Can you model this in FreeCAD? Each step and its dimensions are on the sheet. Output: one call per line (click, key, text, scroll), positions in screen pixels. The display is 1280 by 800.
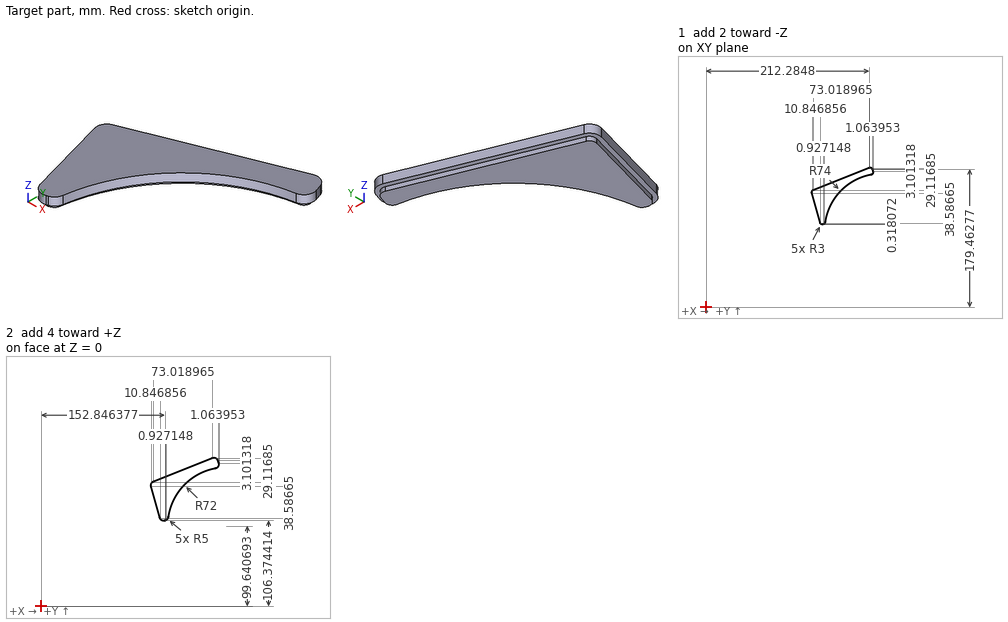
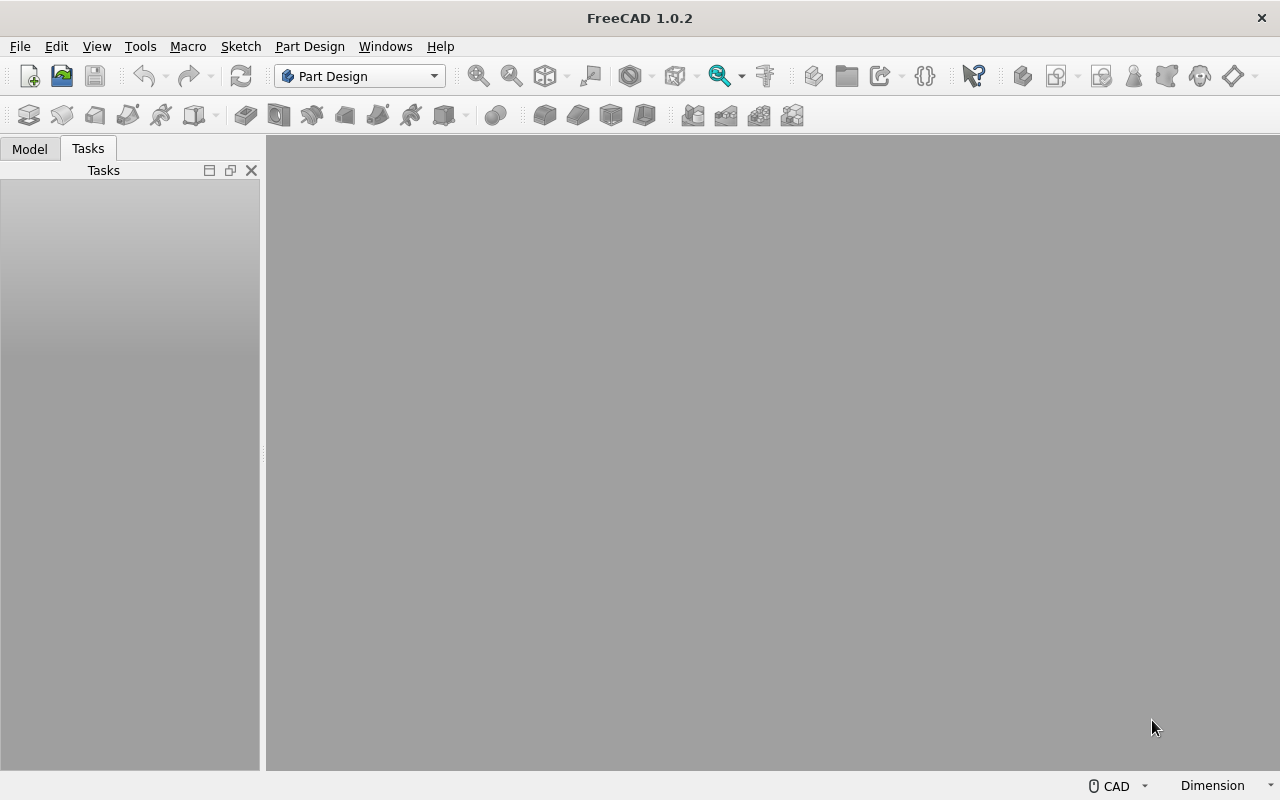
click(29, 76)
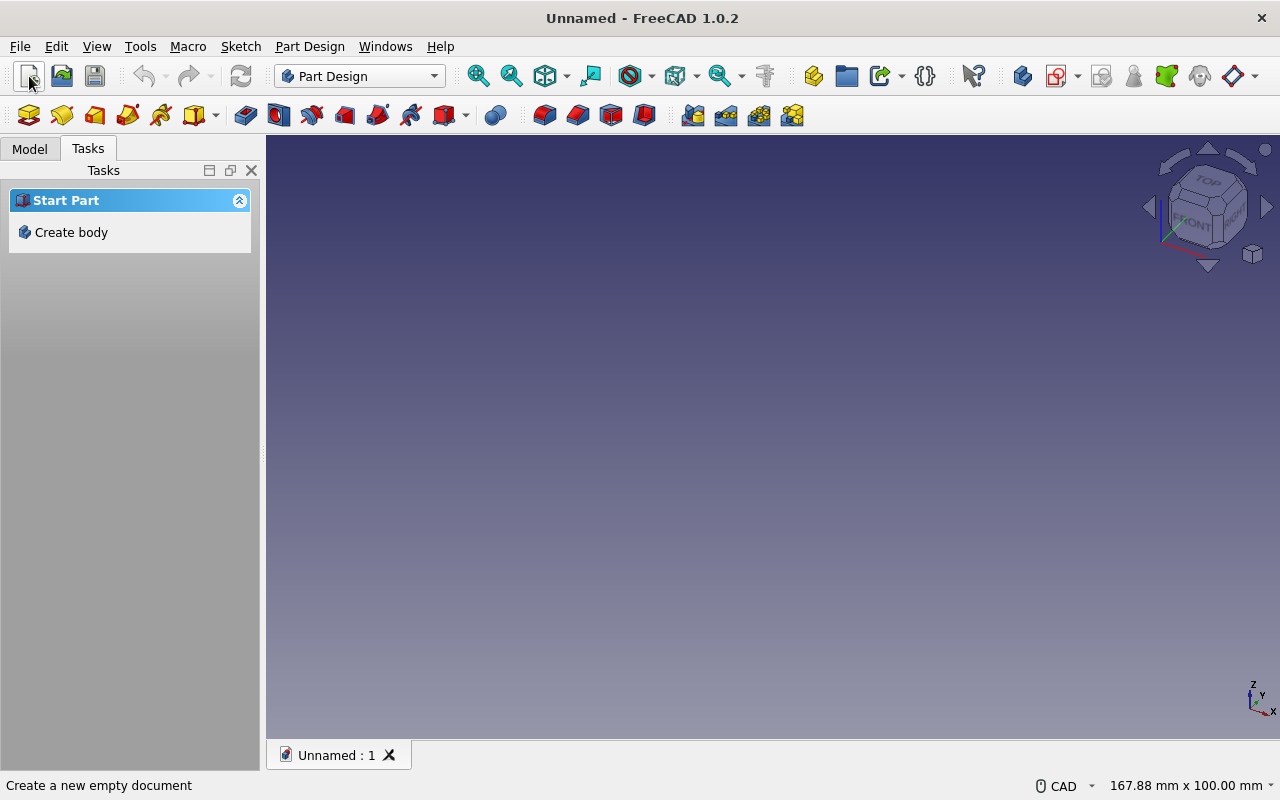
click(1056, 76)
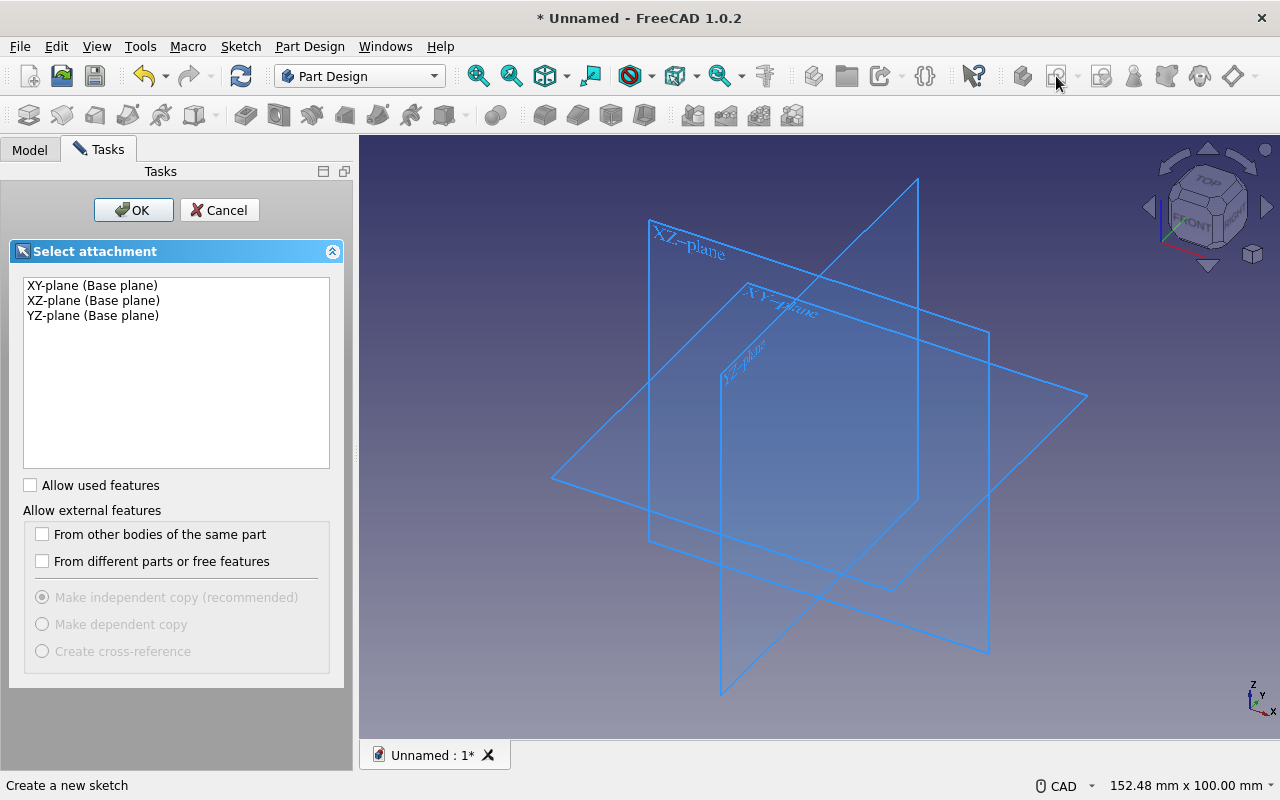
click(84, 286)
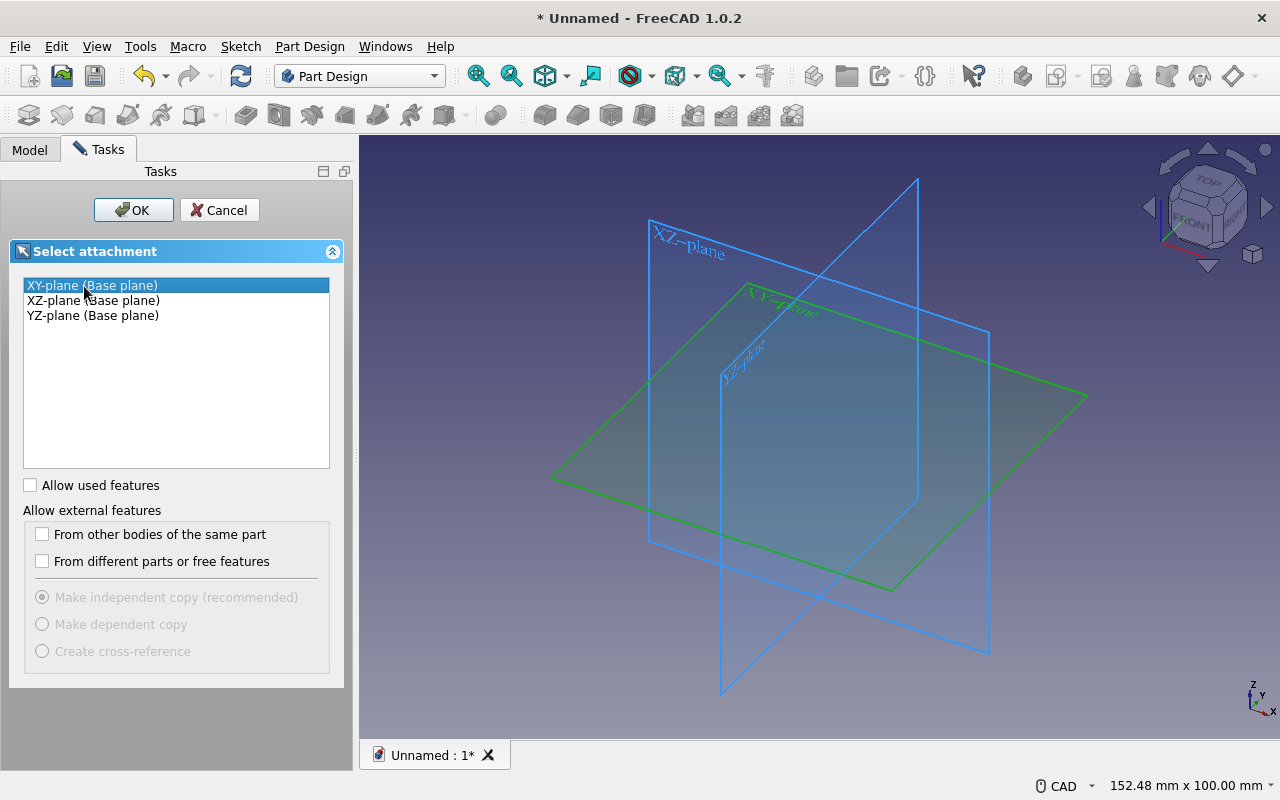
click(134, 210)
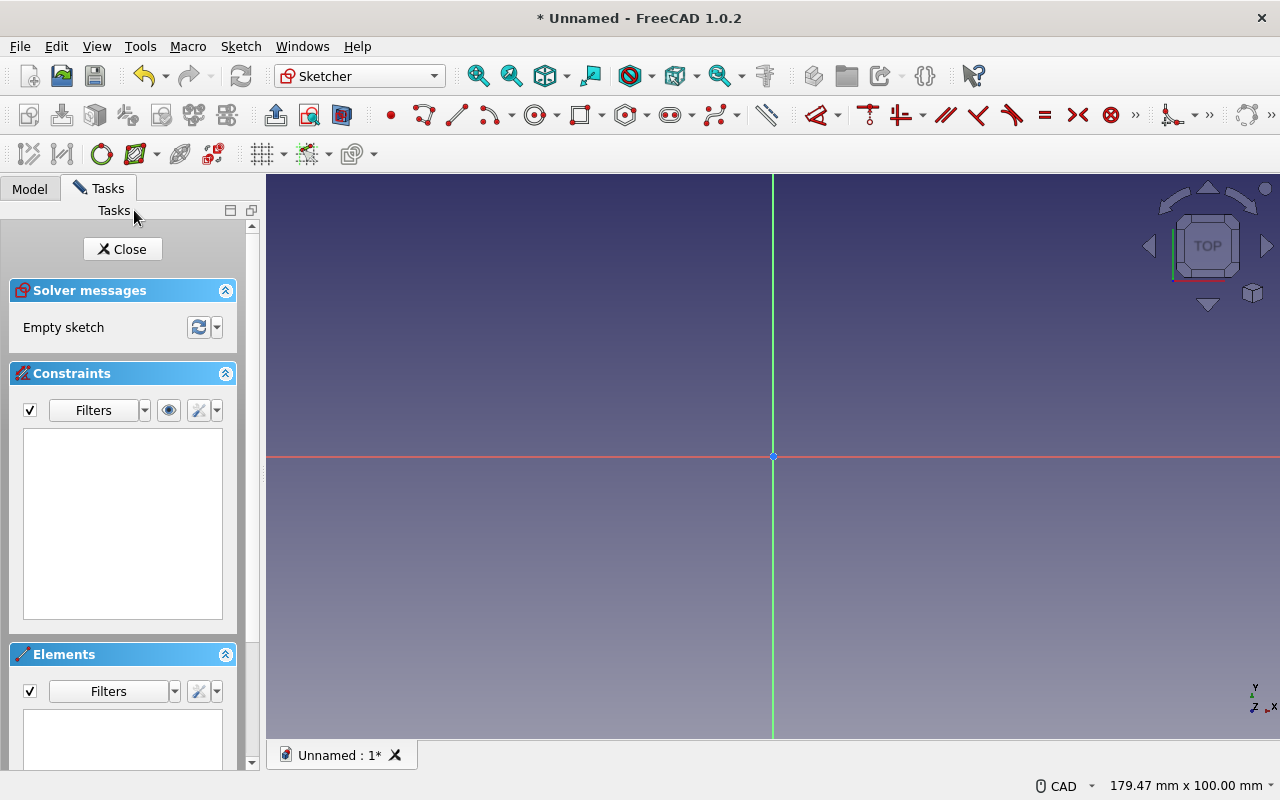
scroll(704, 456, down, 5)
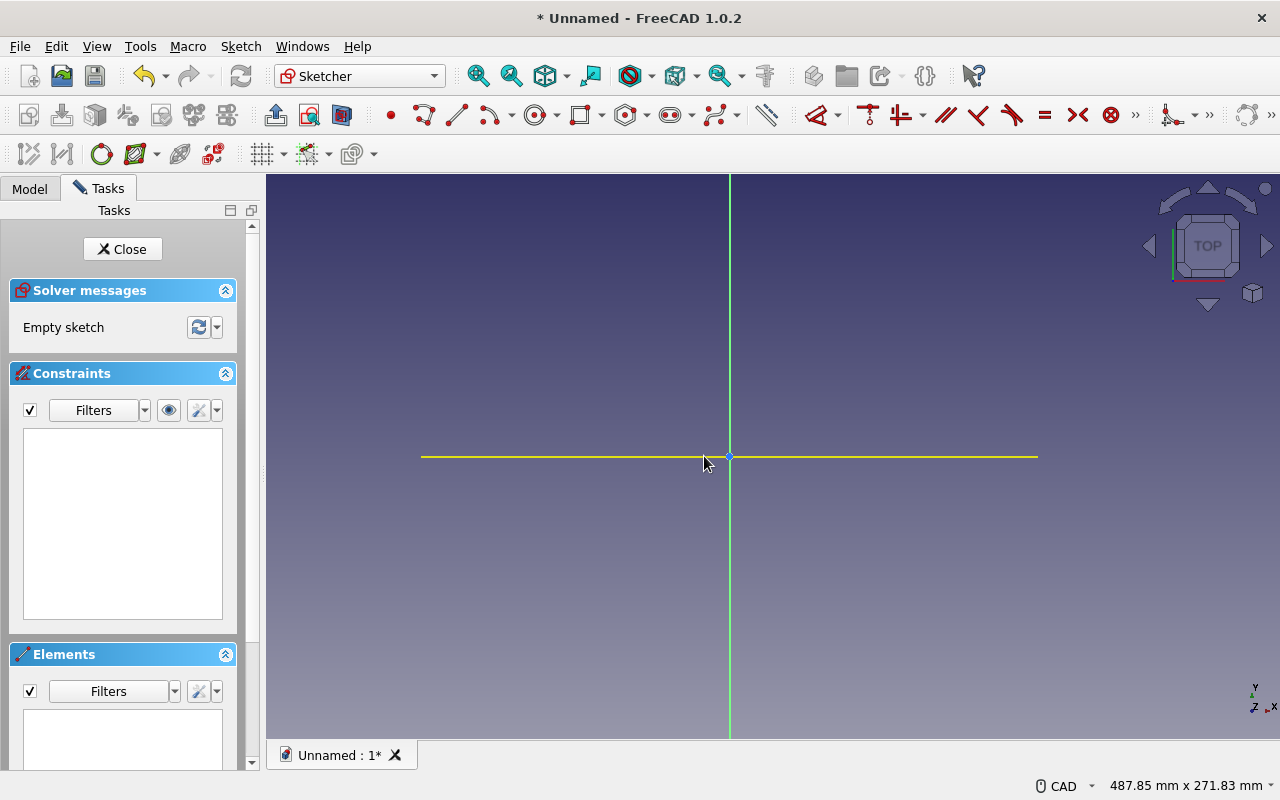
scroll(704, 456, down, 5)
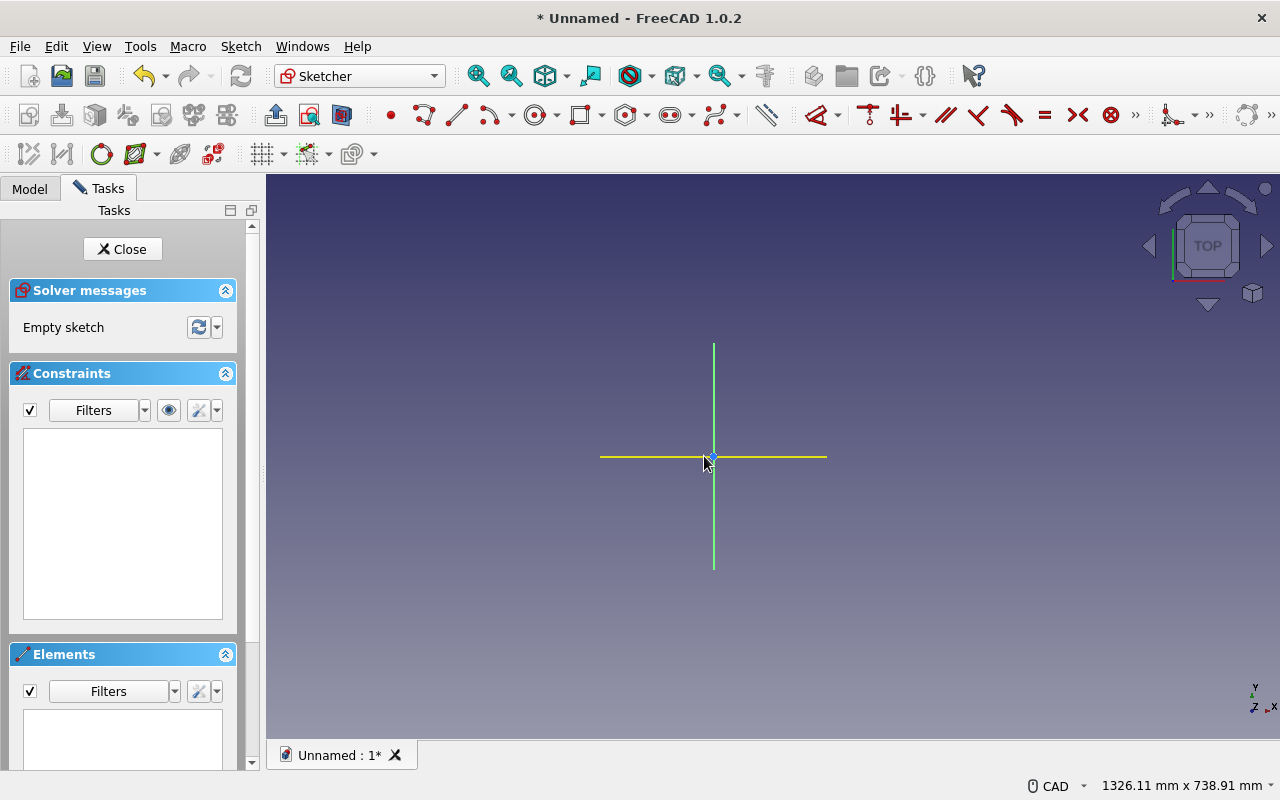
scroll(878, 324, up, 9)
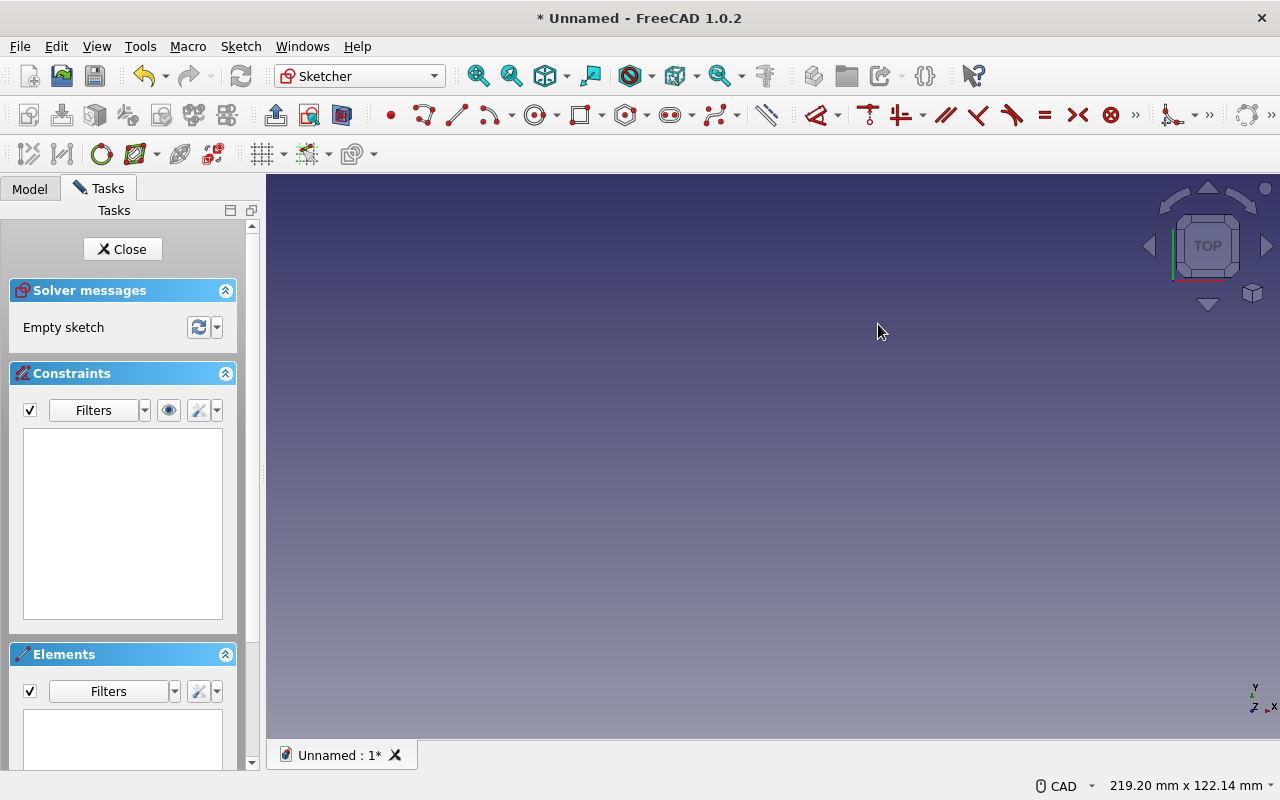
click(457, 116)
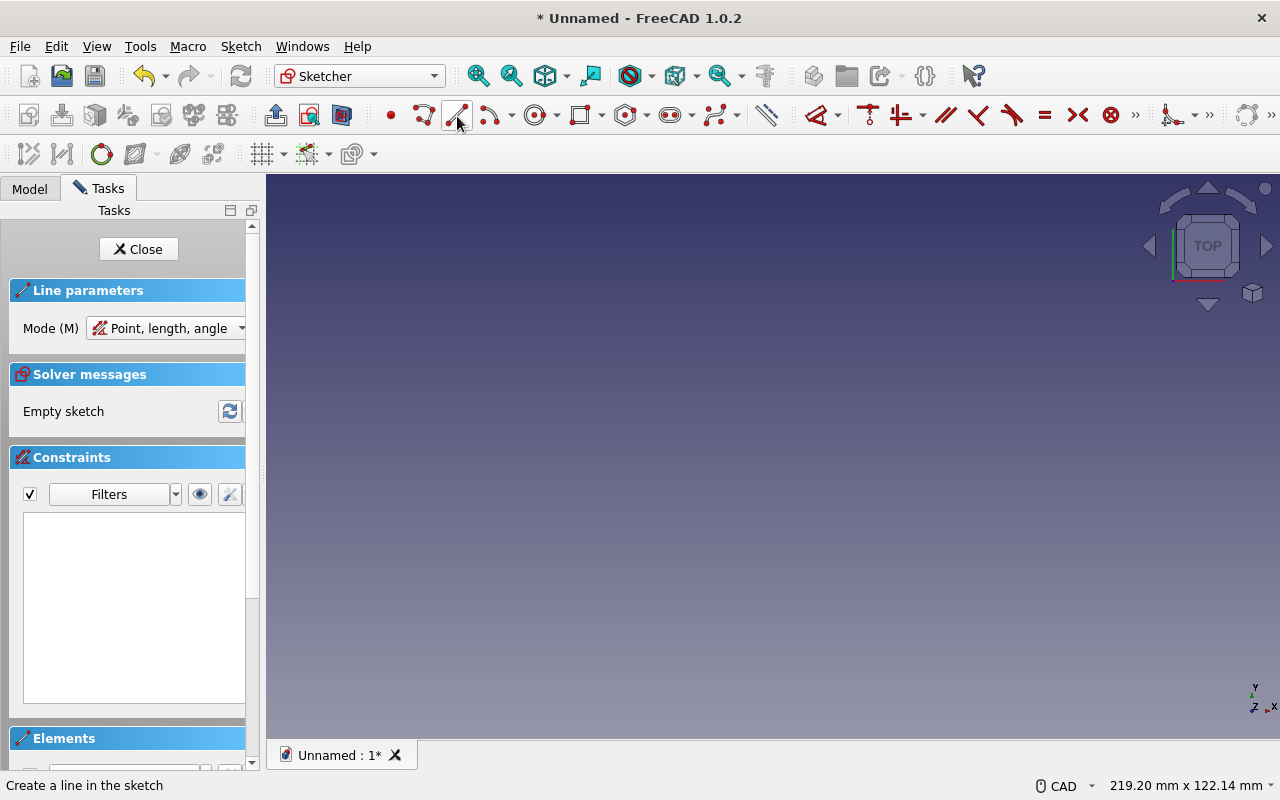
click(517, 437)
click(567, 616)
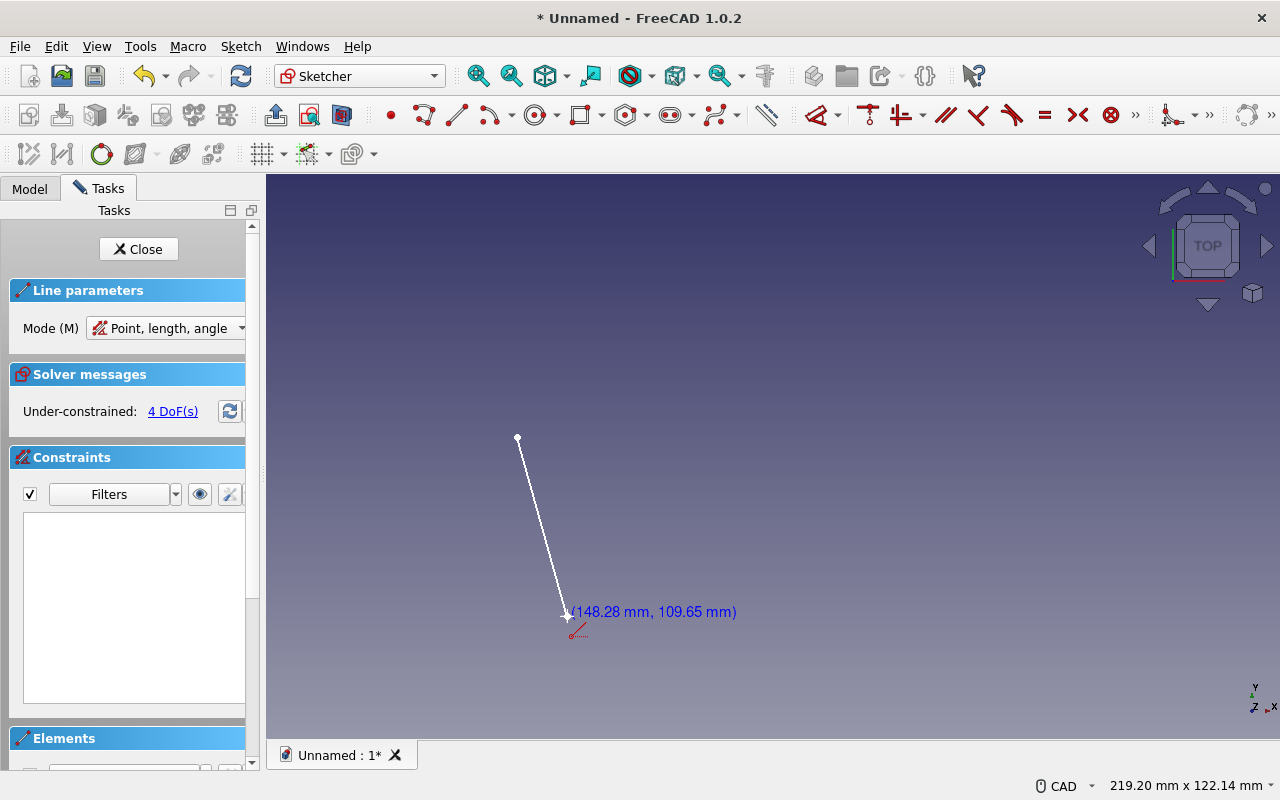
click(585, 625)